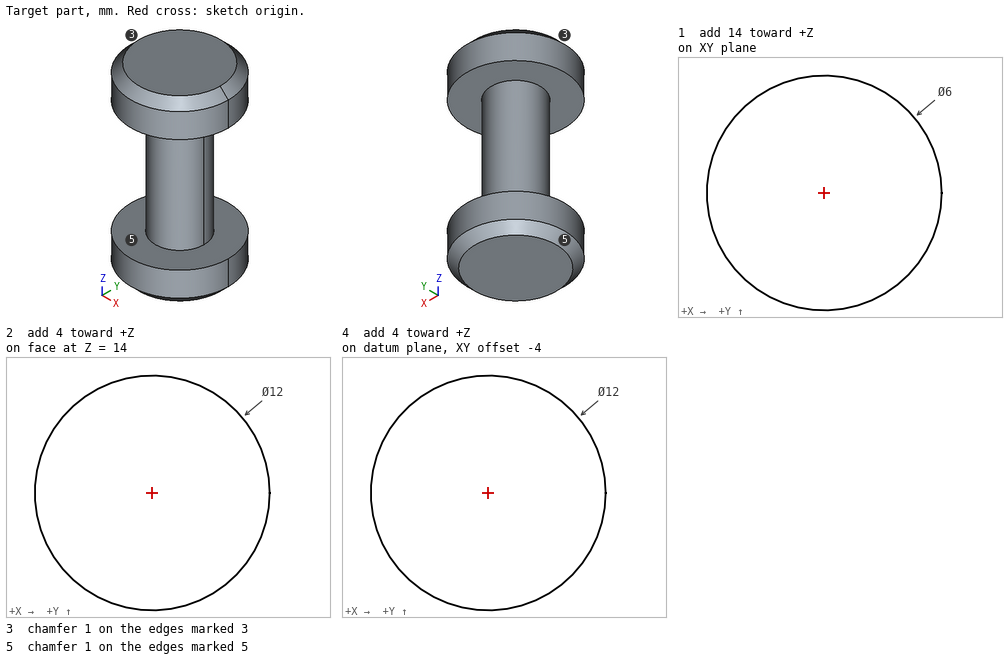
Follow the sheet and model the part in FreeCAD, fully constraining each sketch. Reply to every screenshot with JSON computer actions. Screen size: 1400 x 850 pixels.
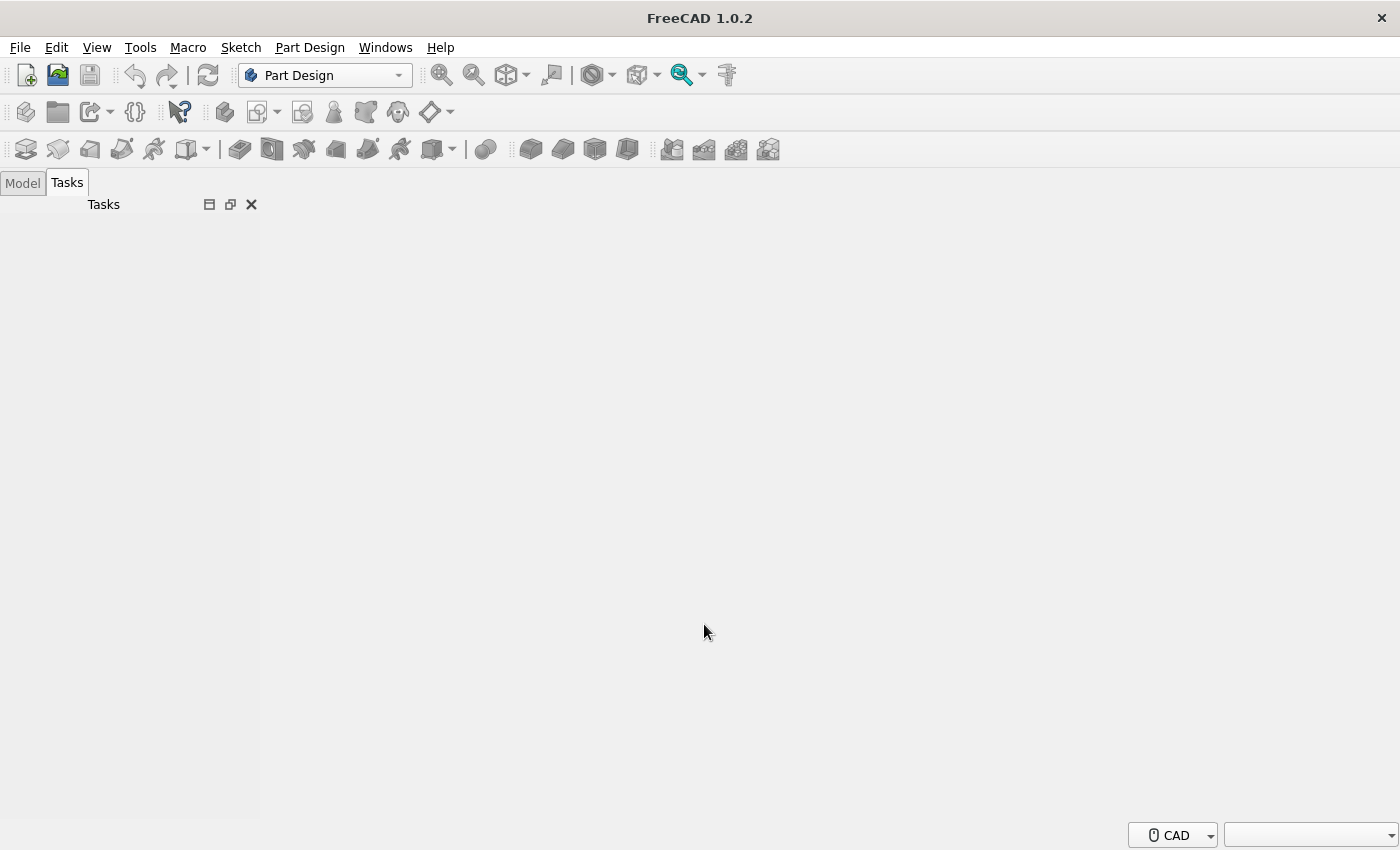
{"action": "key", "text": "ctrl+n"}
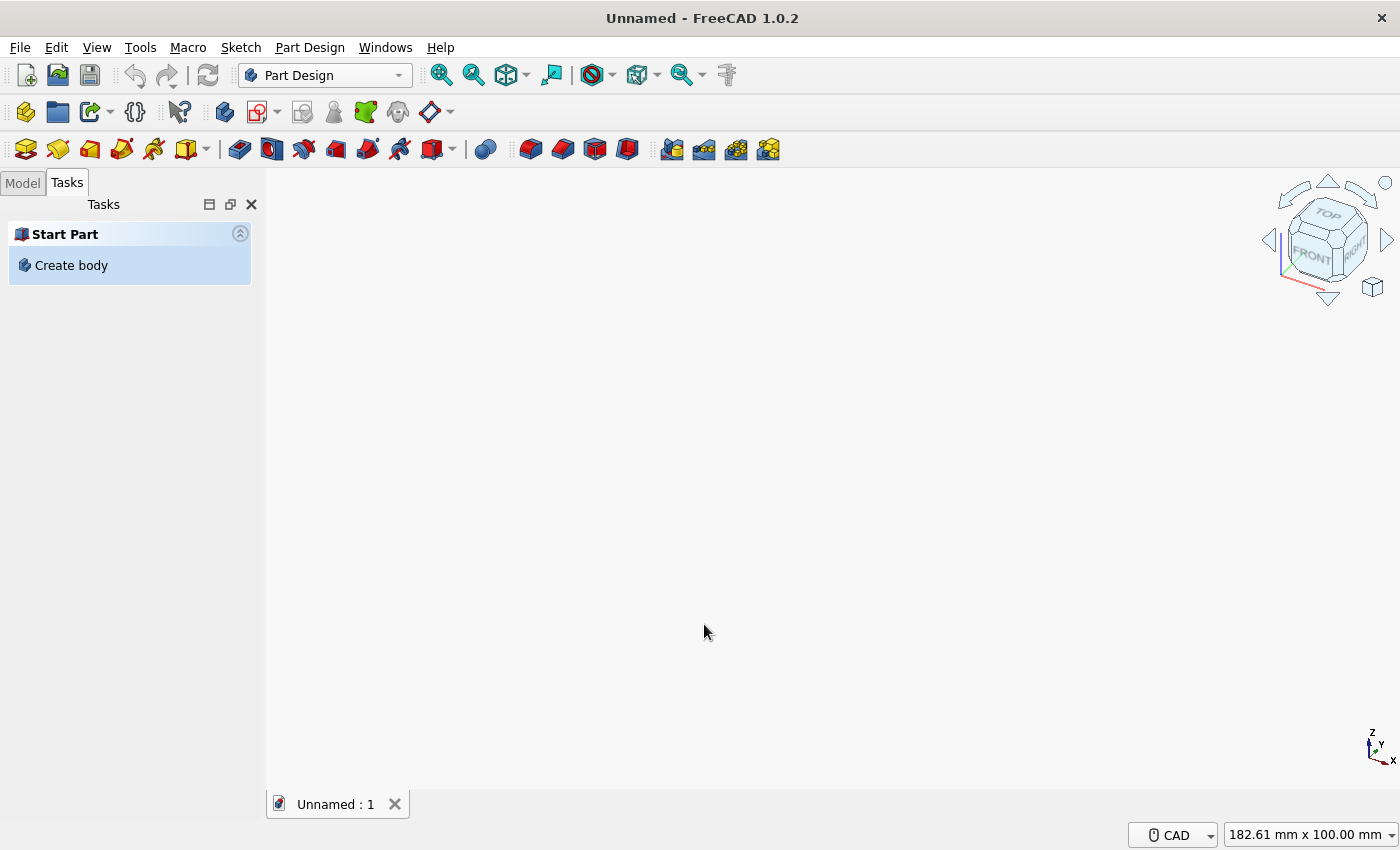
{"action": "left_click", "coordinate": [258, 112]}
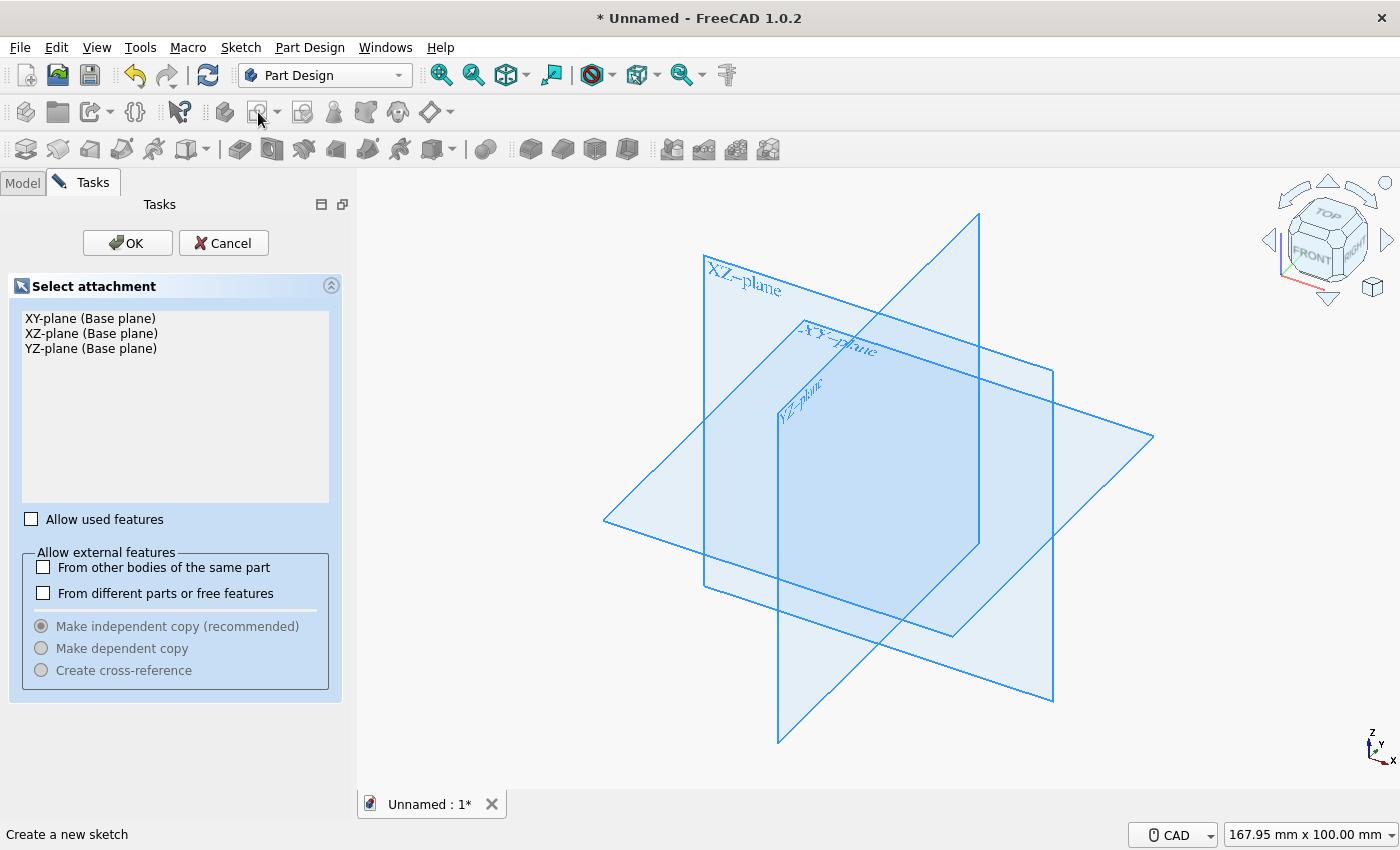
{"action": "left_click", "coordinate": [82, 318]}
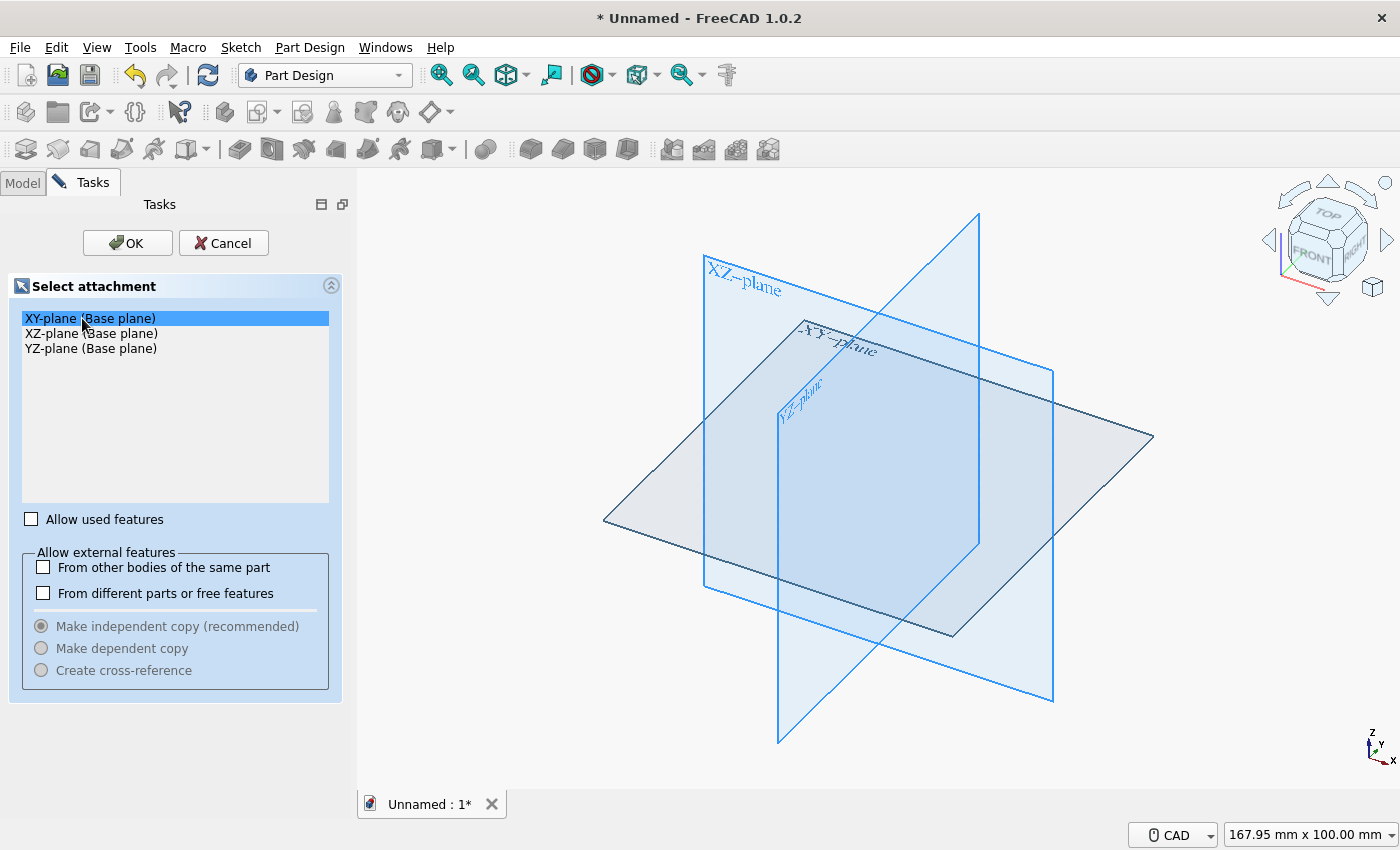
{"action": "left_click", "coordinate": [128, 243]}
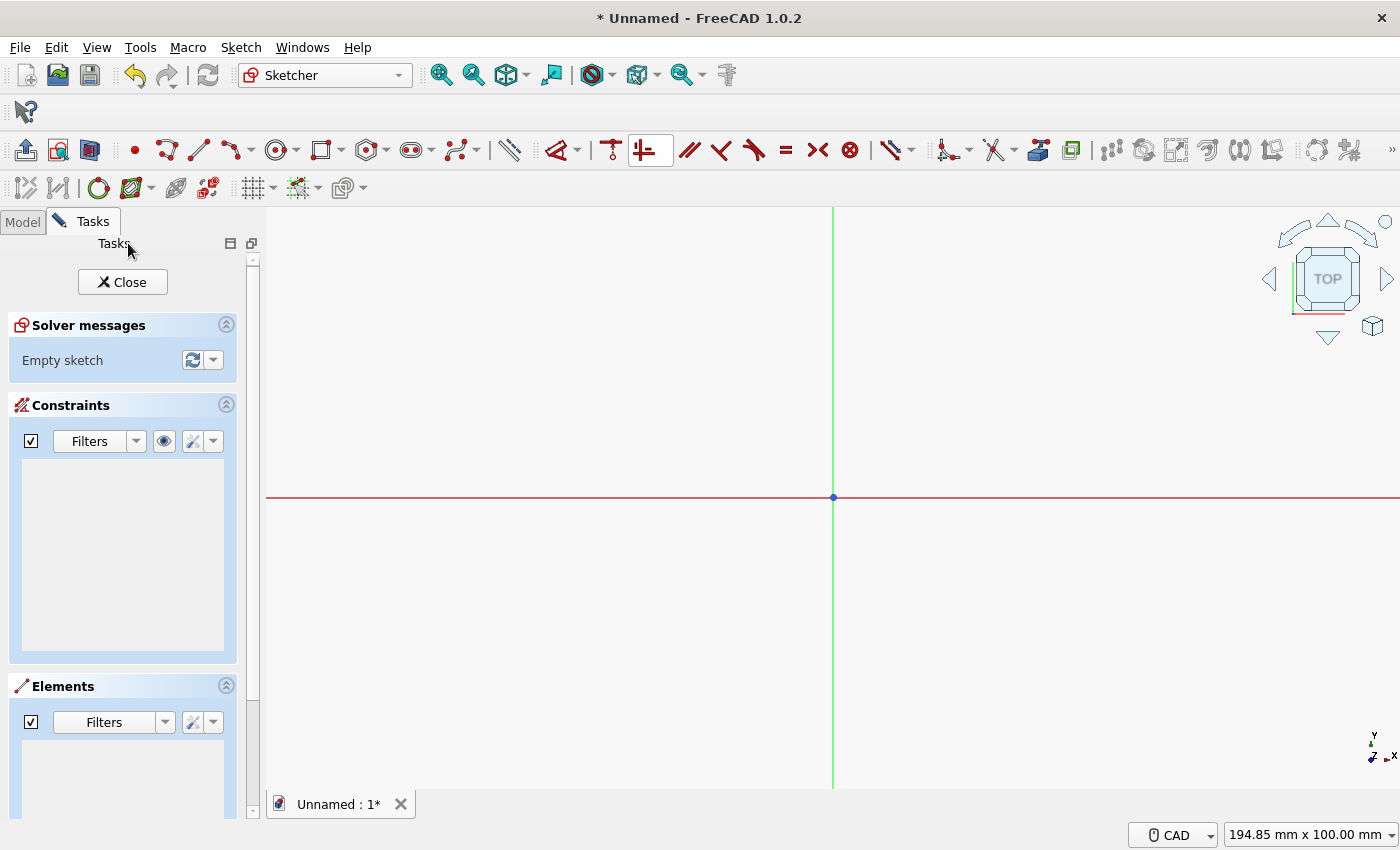
{"action": "scroll", "coordinate": [840, 498], "scroll_direction": "up", "scroll_amount": 12}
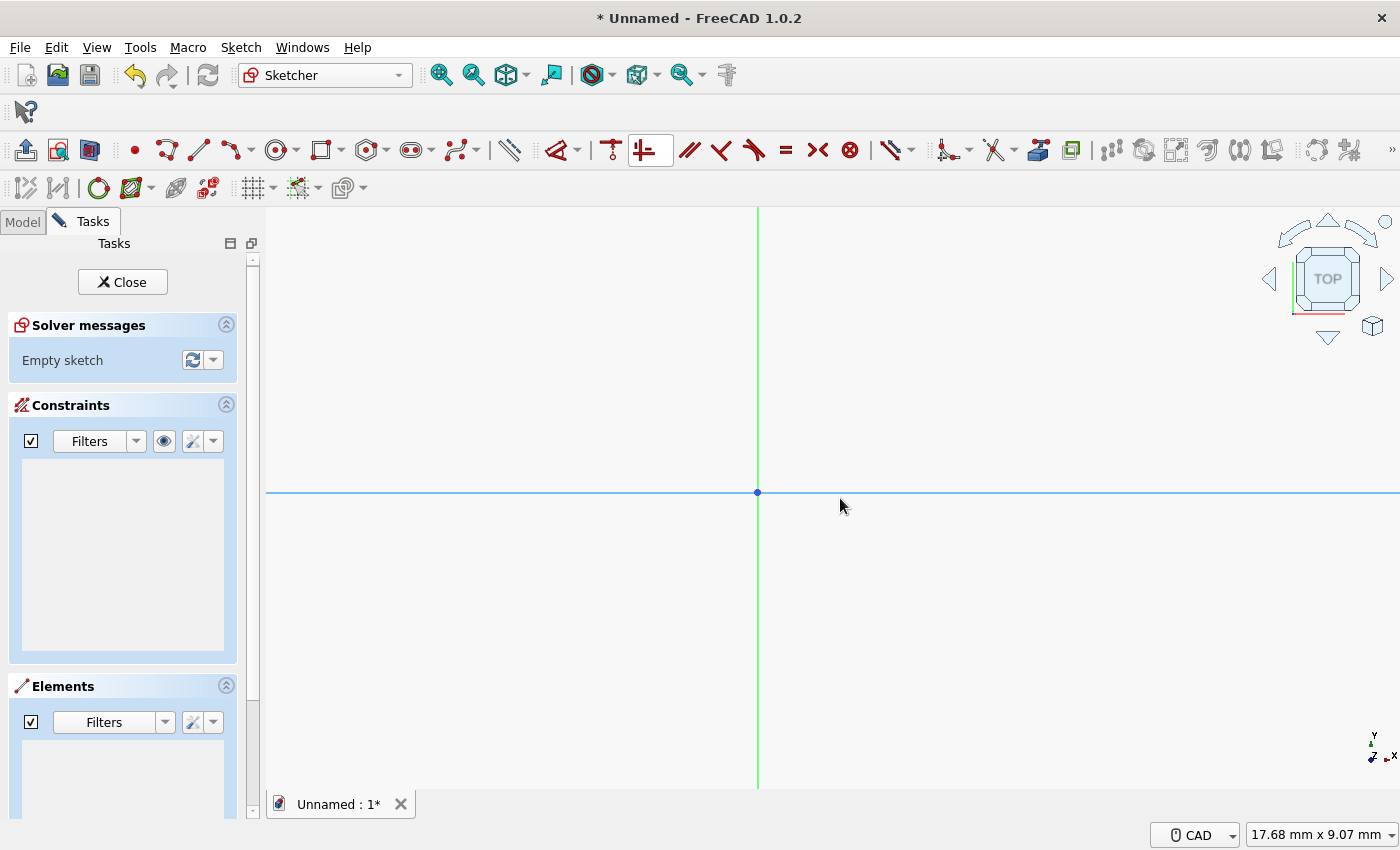
{"action": "key", "text": "g c"}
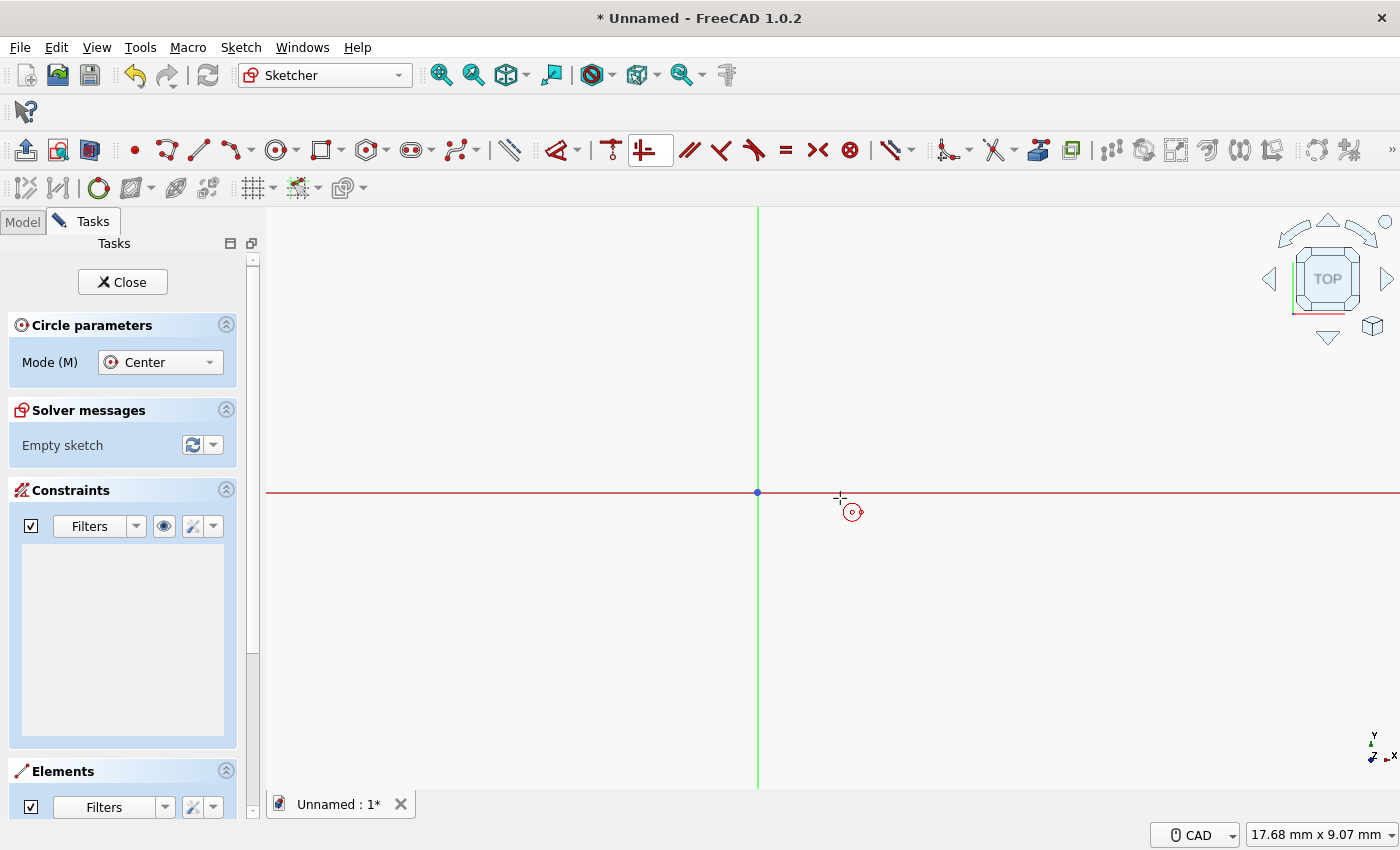
{"action": "left_click", "coordinate": [758, 493]}
{"action": "left_click", "coordinate": [894, 357]}
{"action": "key", "text": "Escape"}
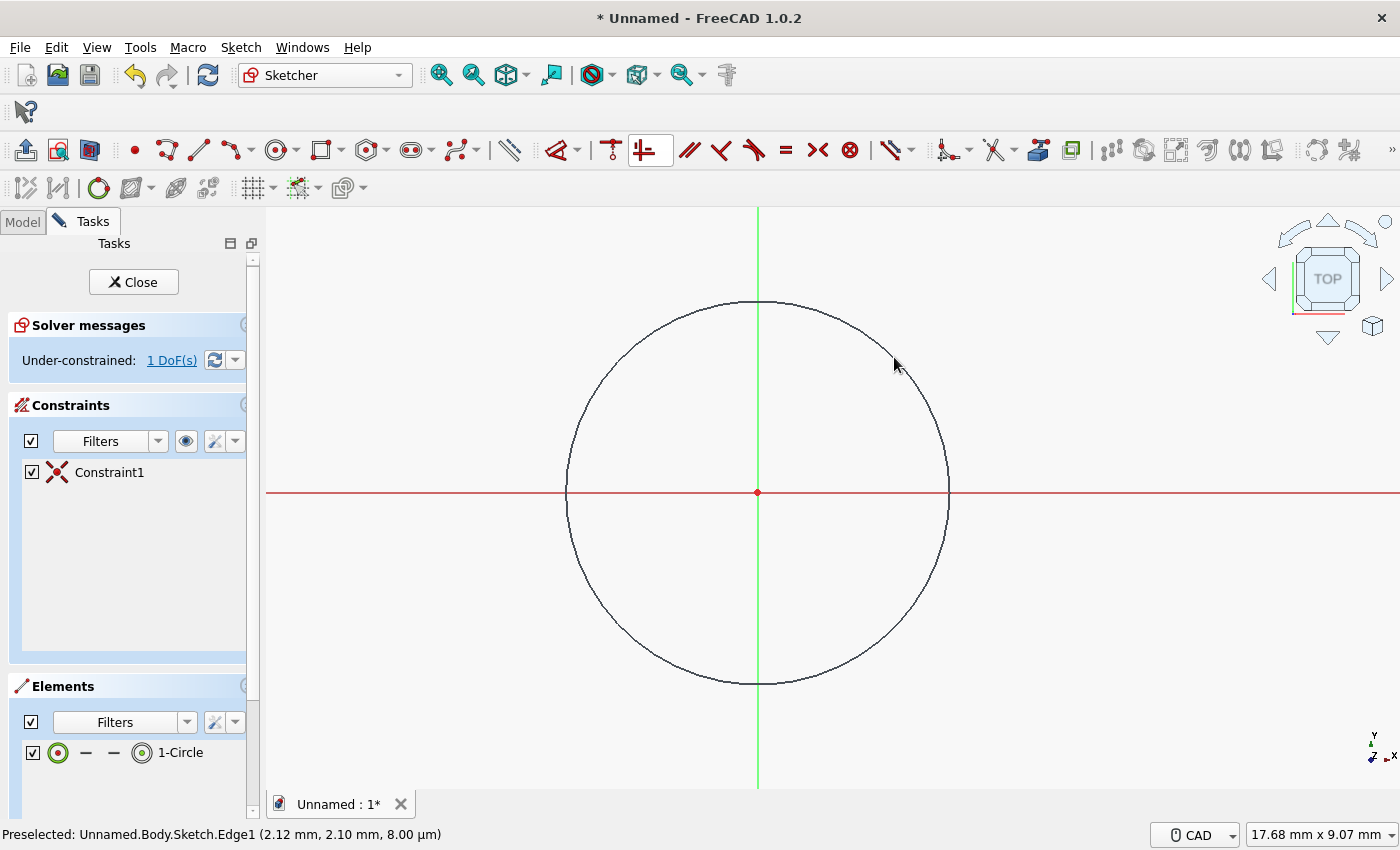
{"action": "left_click", "coordinate": [893, 357]}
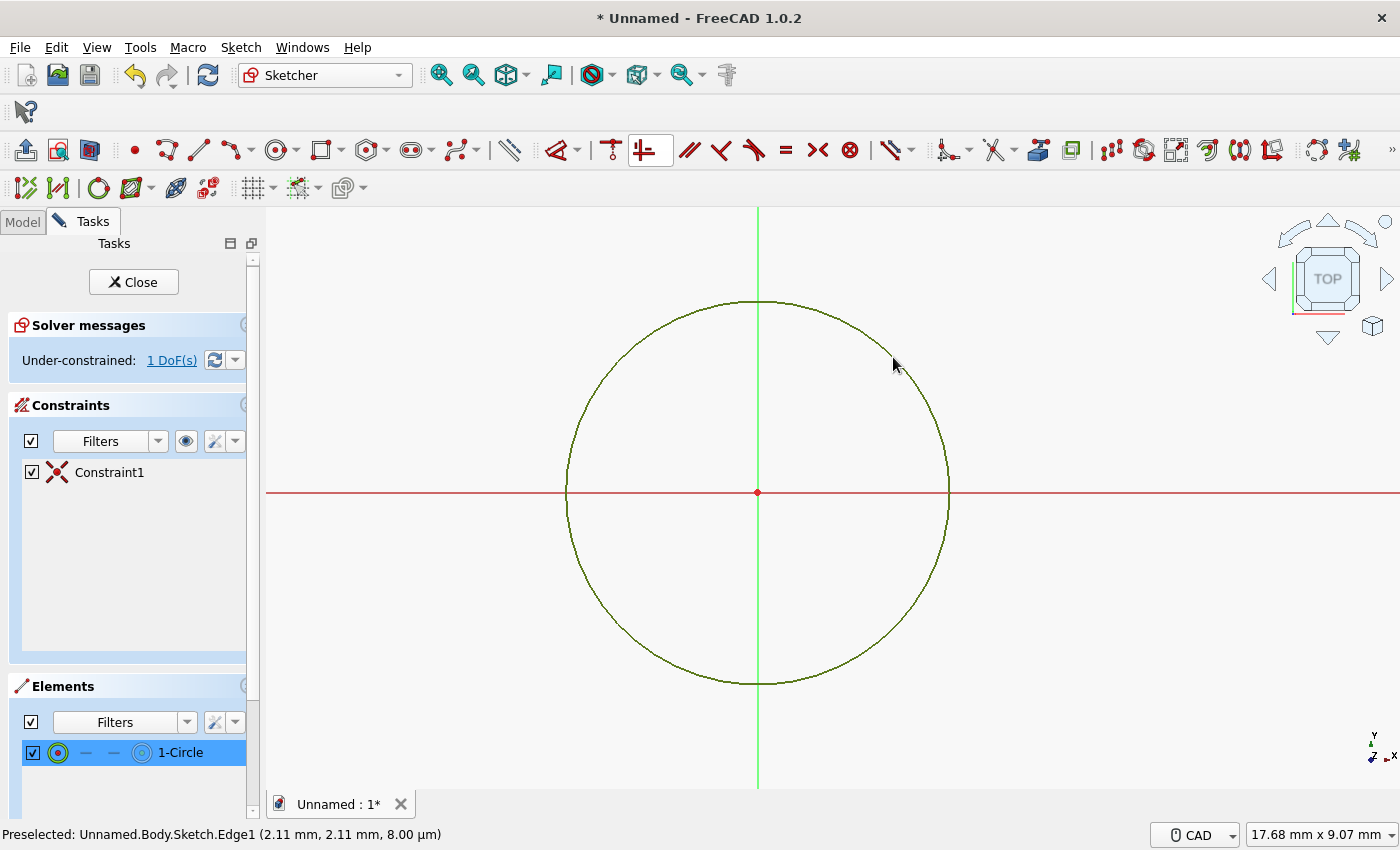
{"action": "key", "text": "k o"}